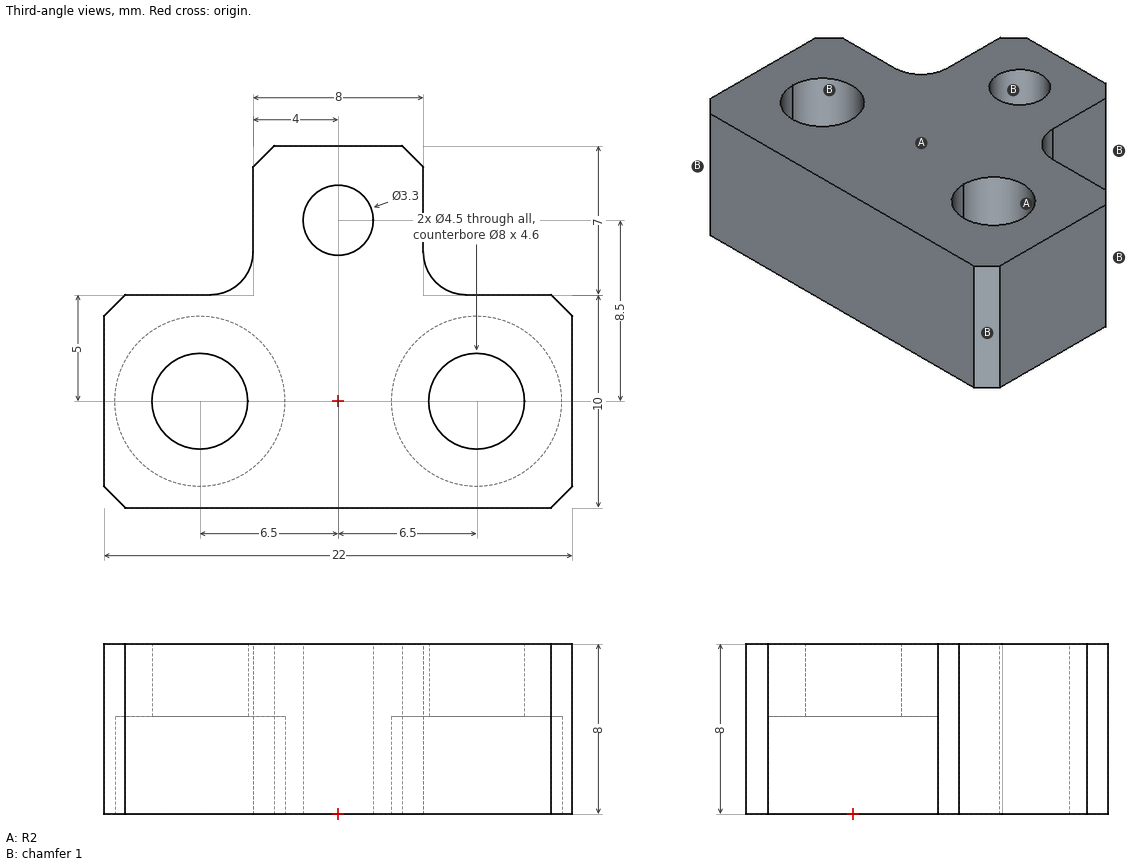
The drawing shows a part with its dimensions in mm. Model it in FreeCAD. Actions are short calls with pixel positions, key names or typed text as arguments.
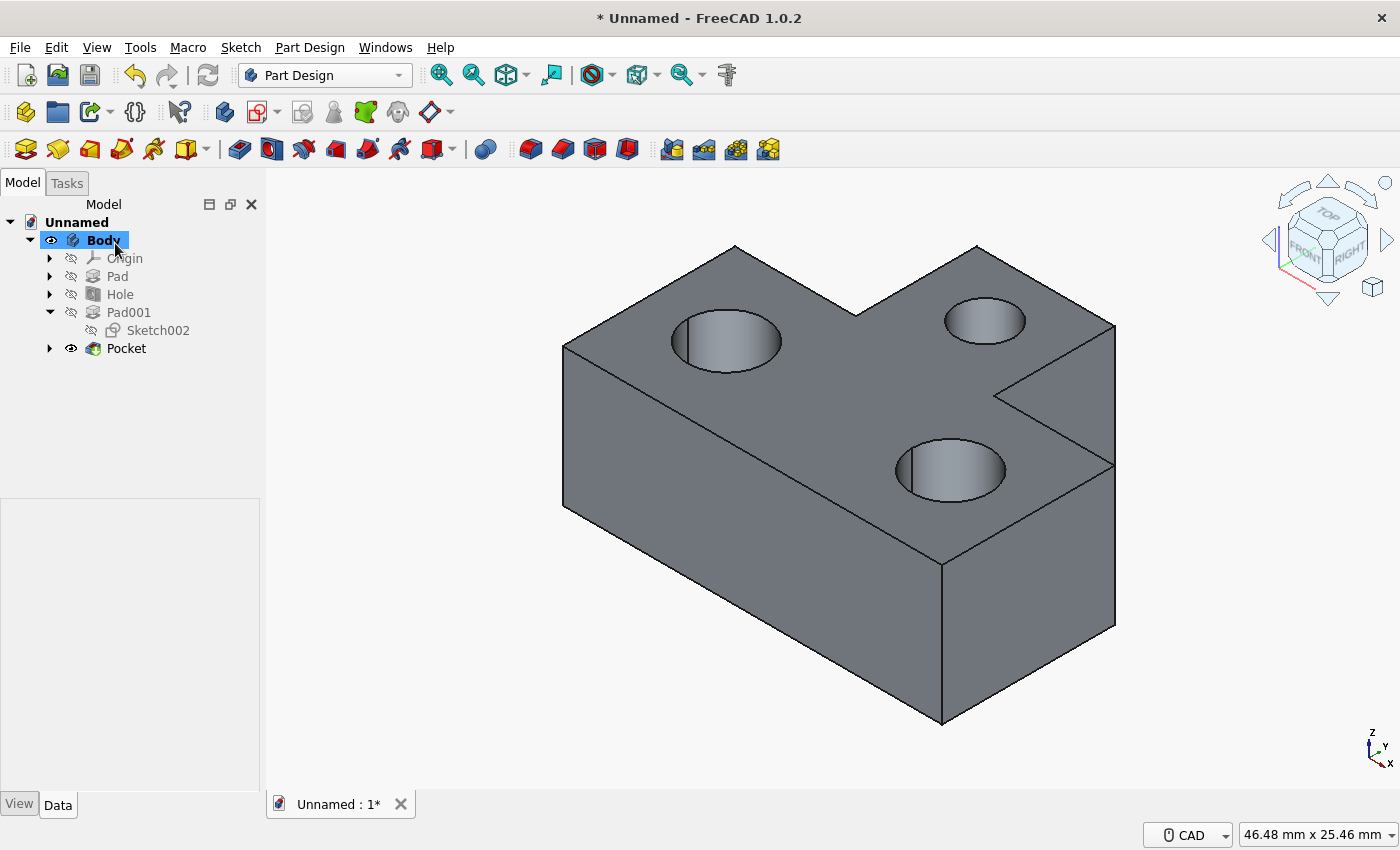
key(2)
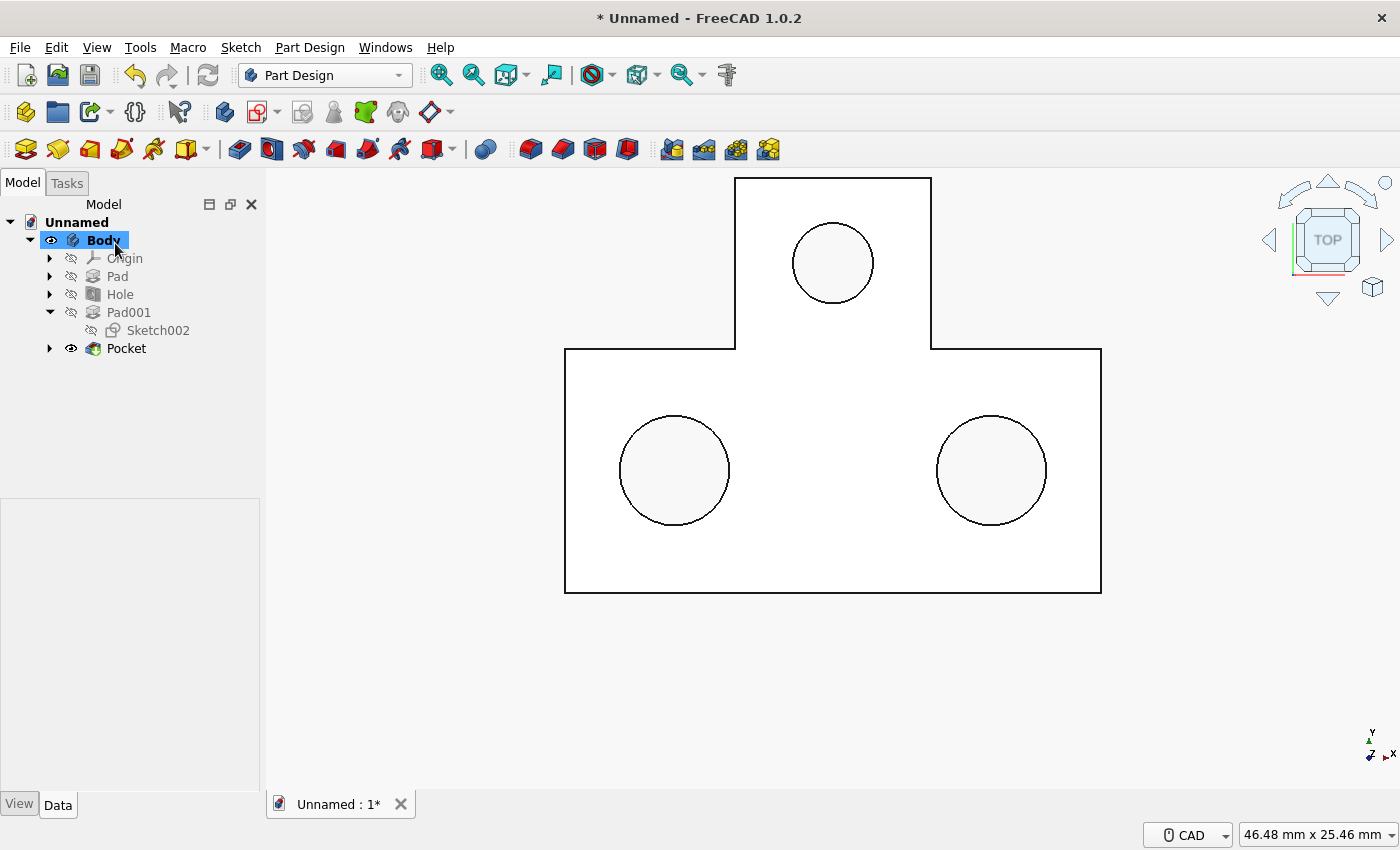
key(1)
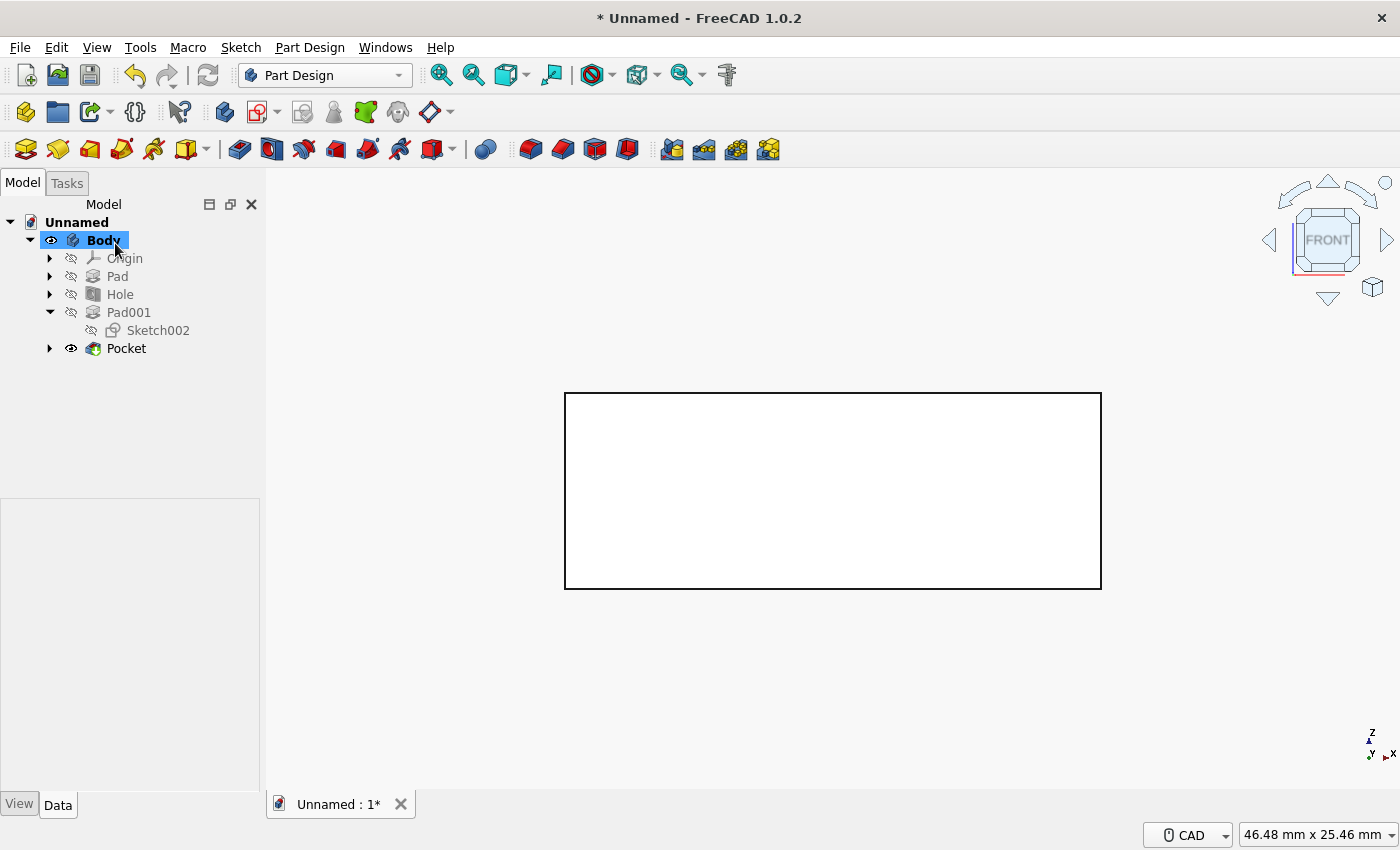
key(3)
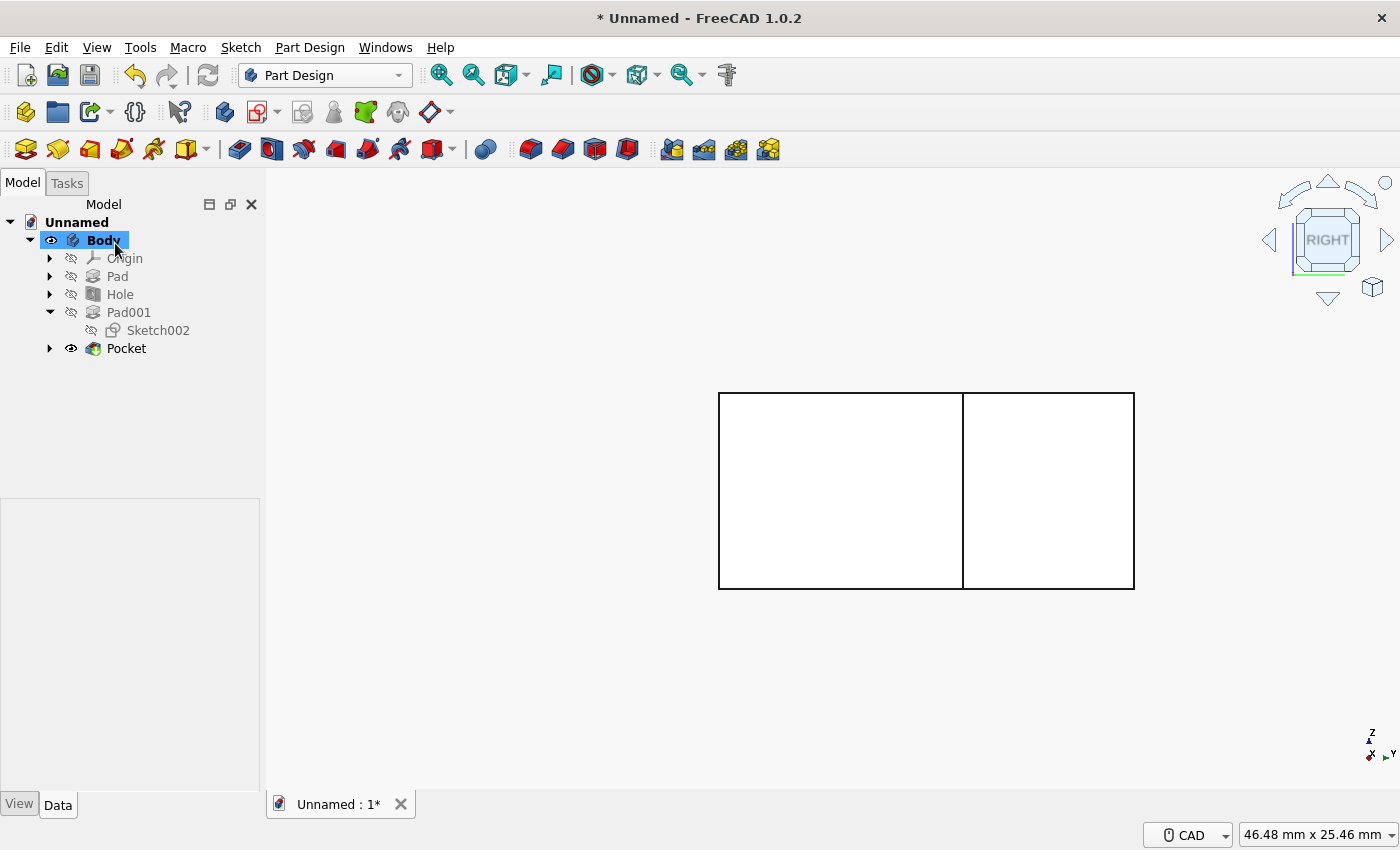
click(442, 76)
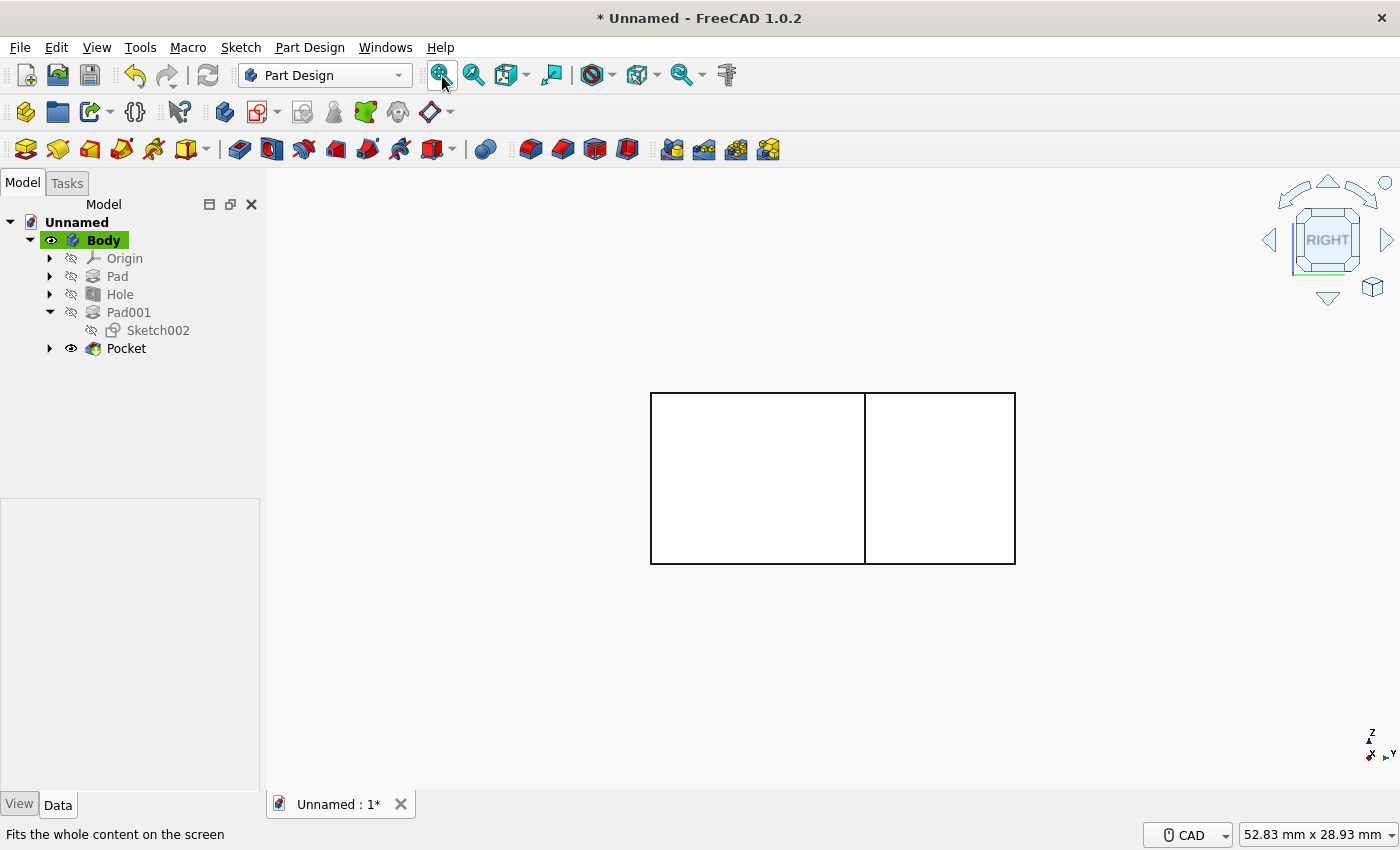
key(5)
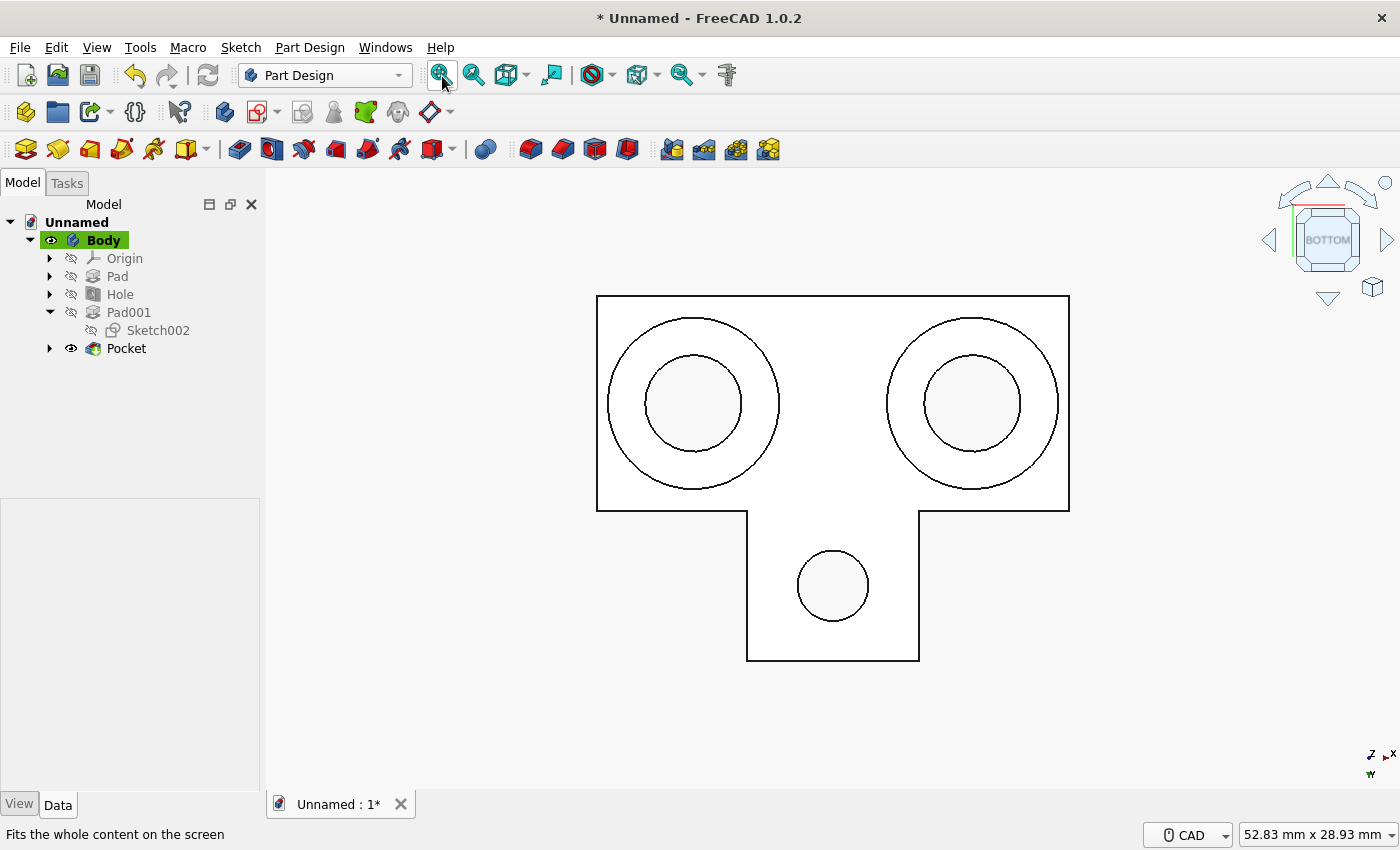
key(4)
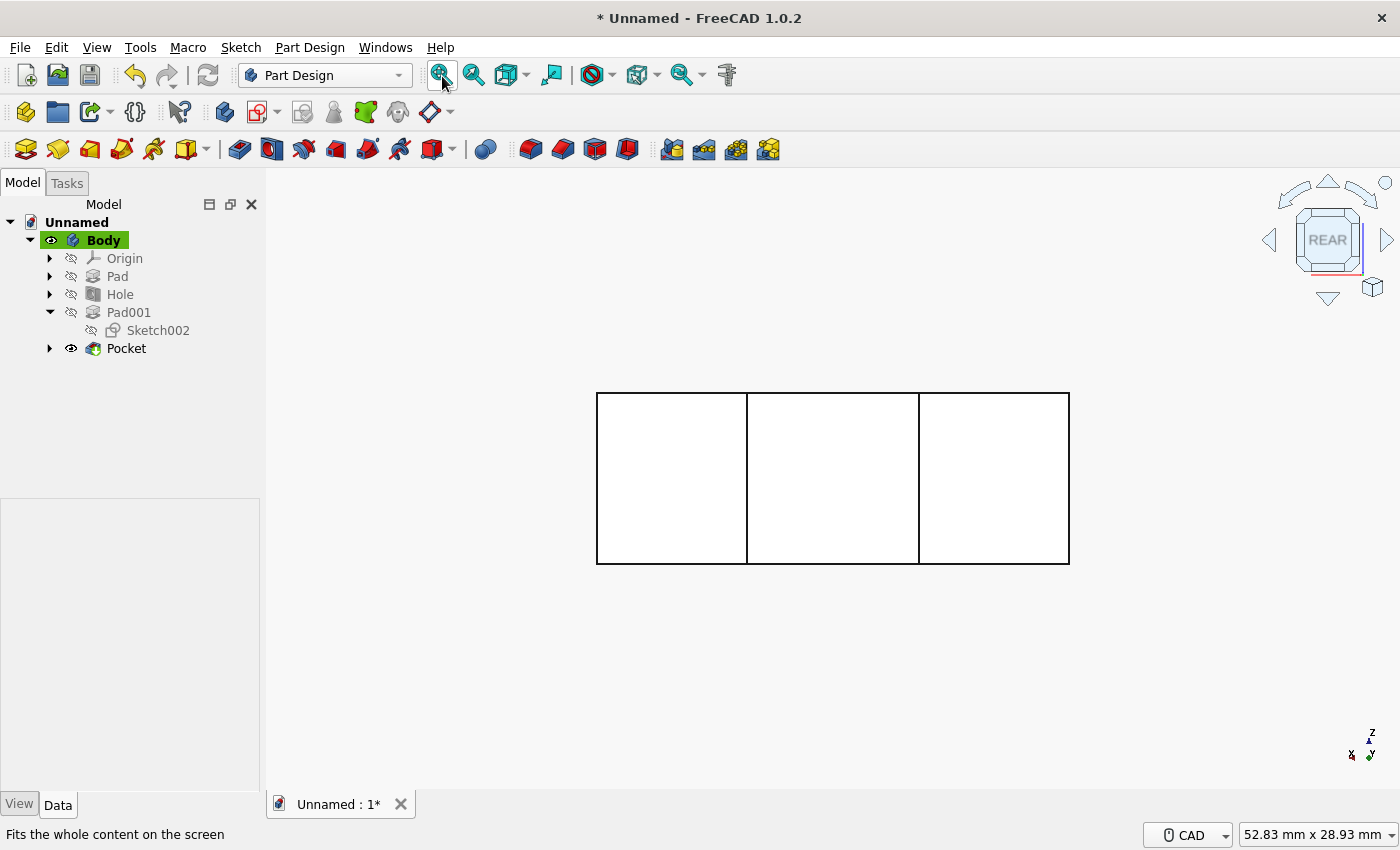
click(442, 76)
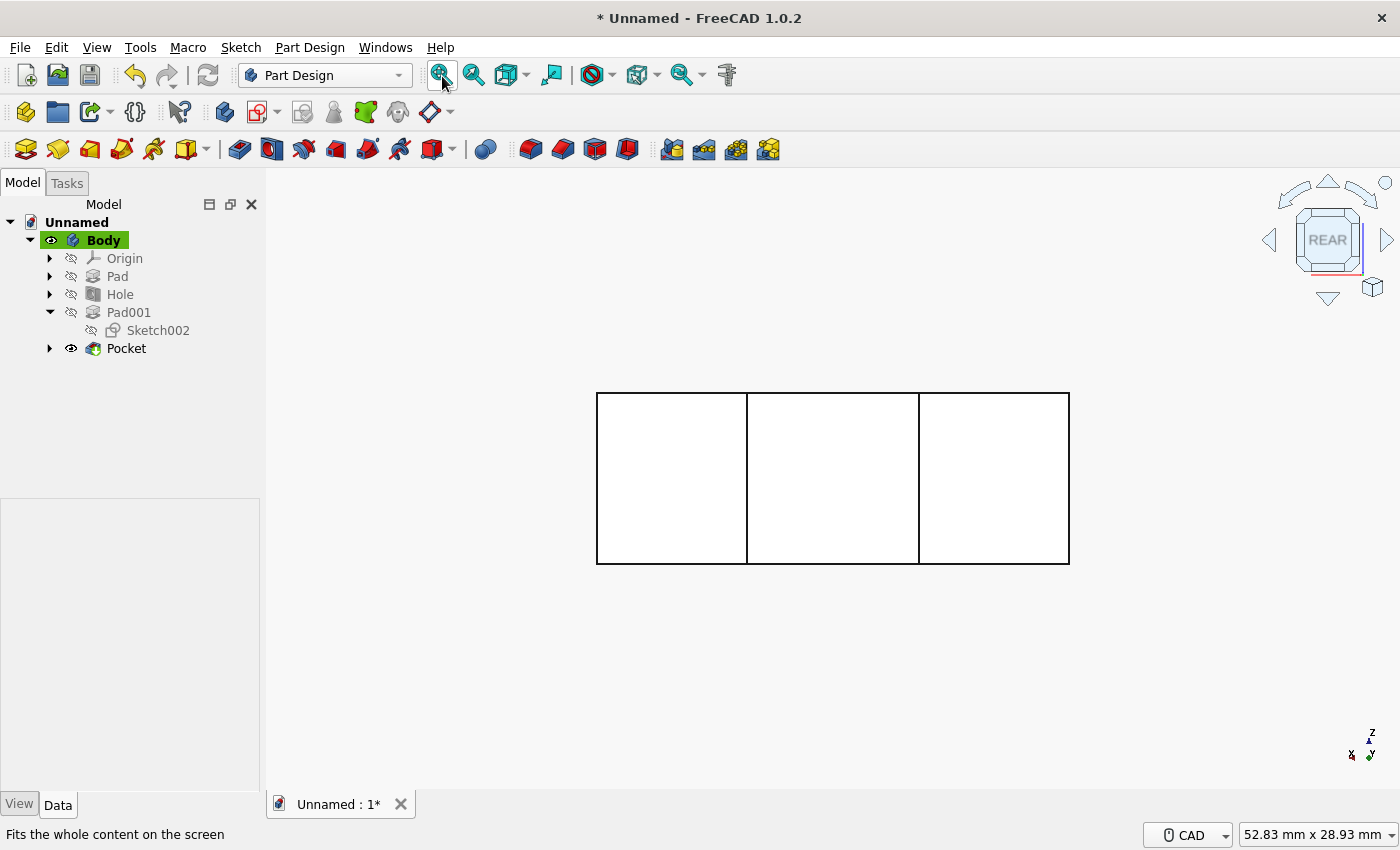
key(6)